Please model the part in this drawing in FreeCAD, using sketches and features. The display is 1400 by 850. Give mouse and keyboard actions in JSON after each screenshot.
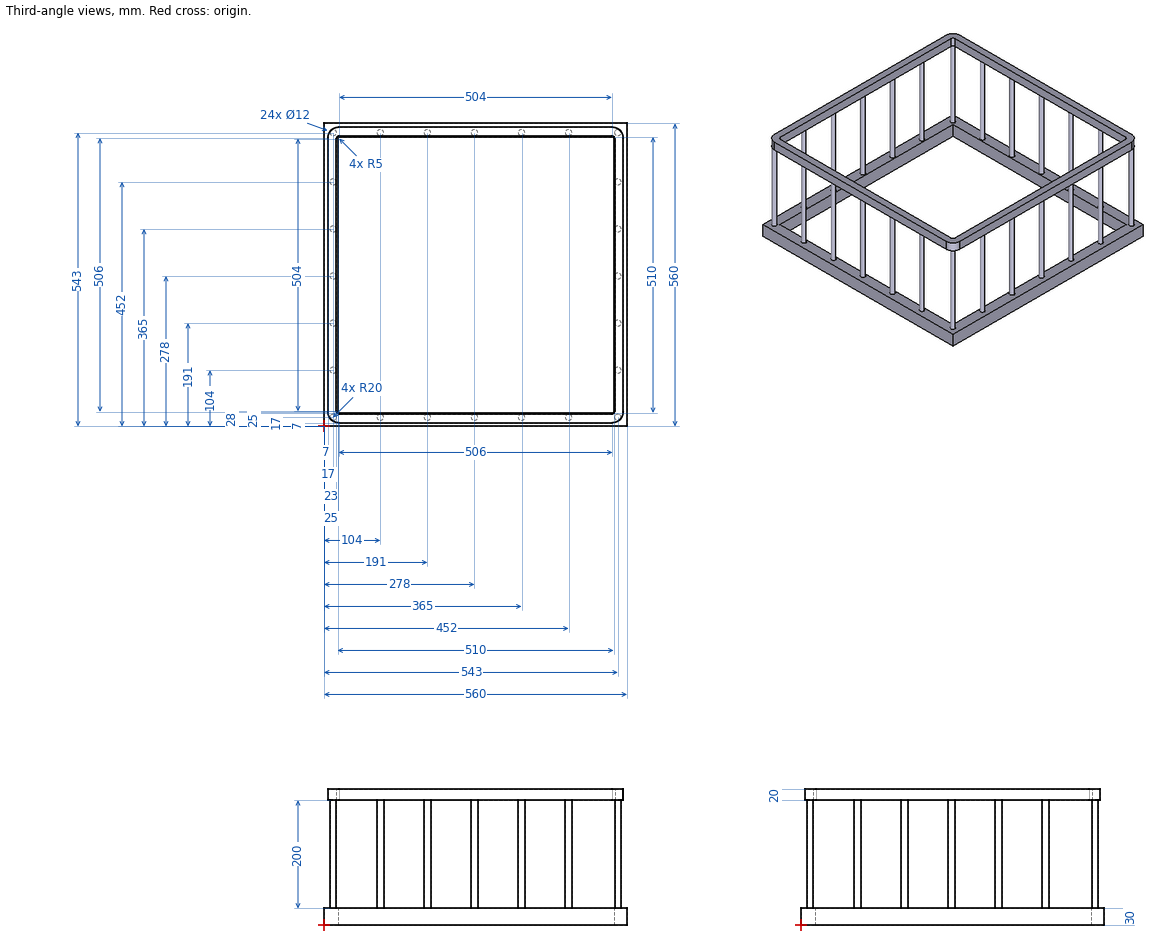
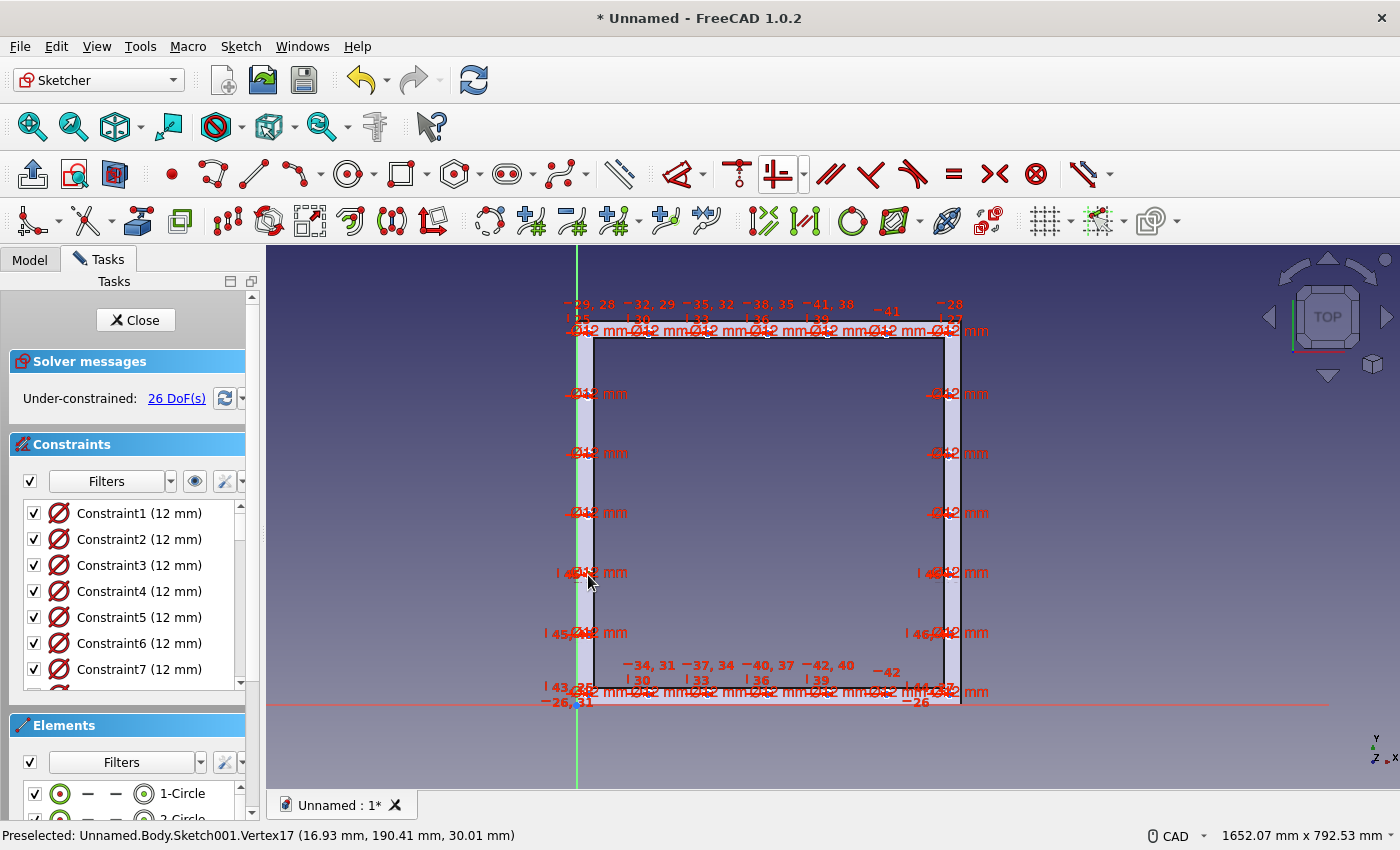
{"action": "left_click", "coordinate": [588, 515]}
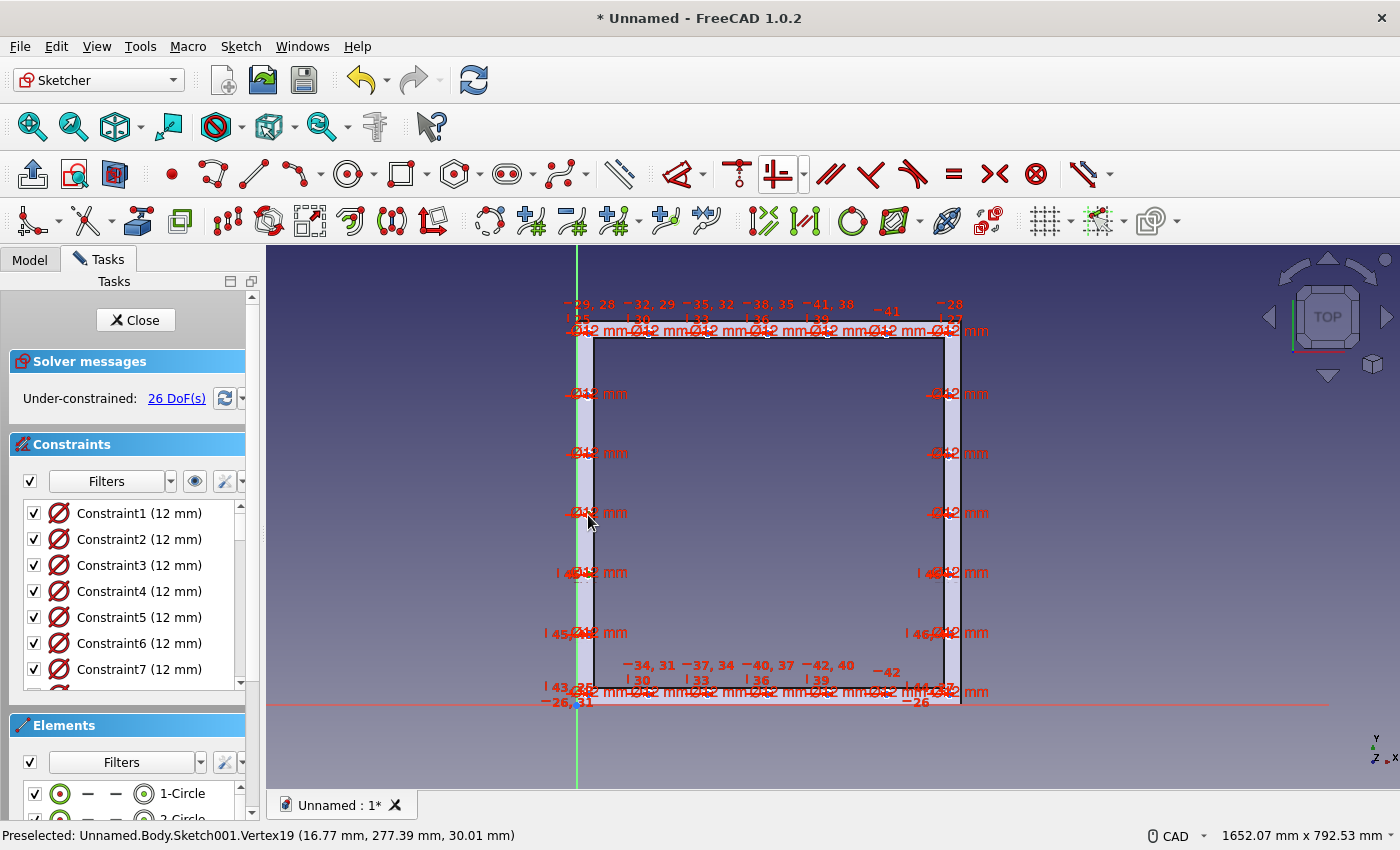
{"action": "key", "text": "v"}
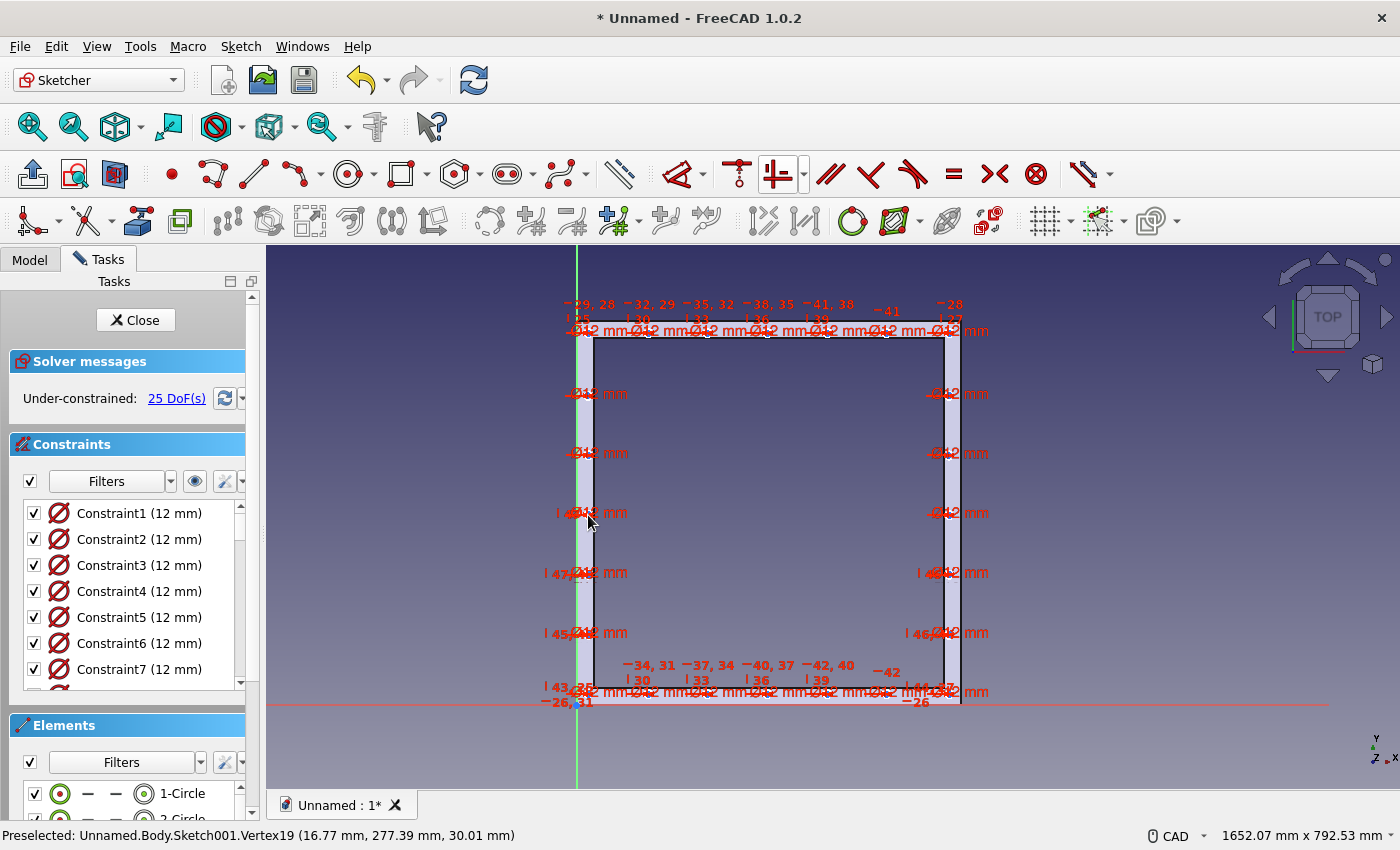
{"action": "left_click", "coordinate": [949, 575]}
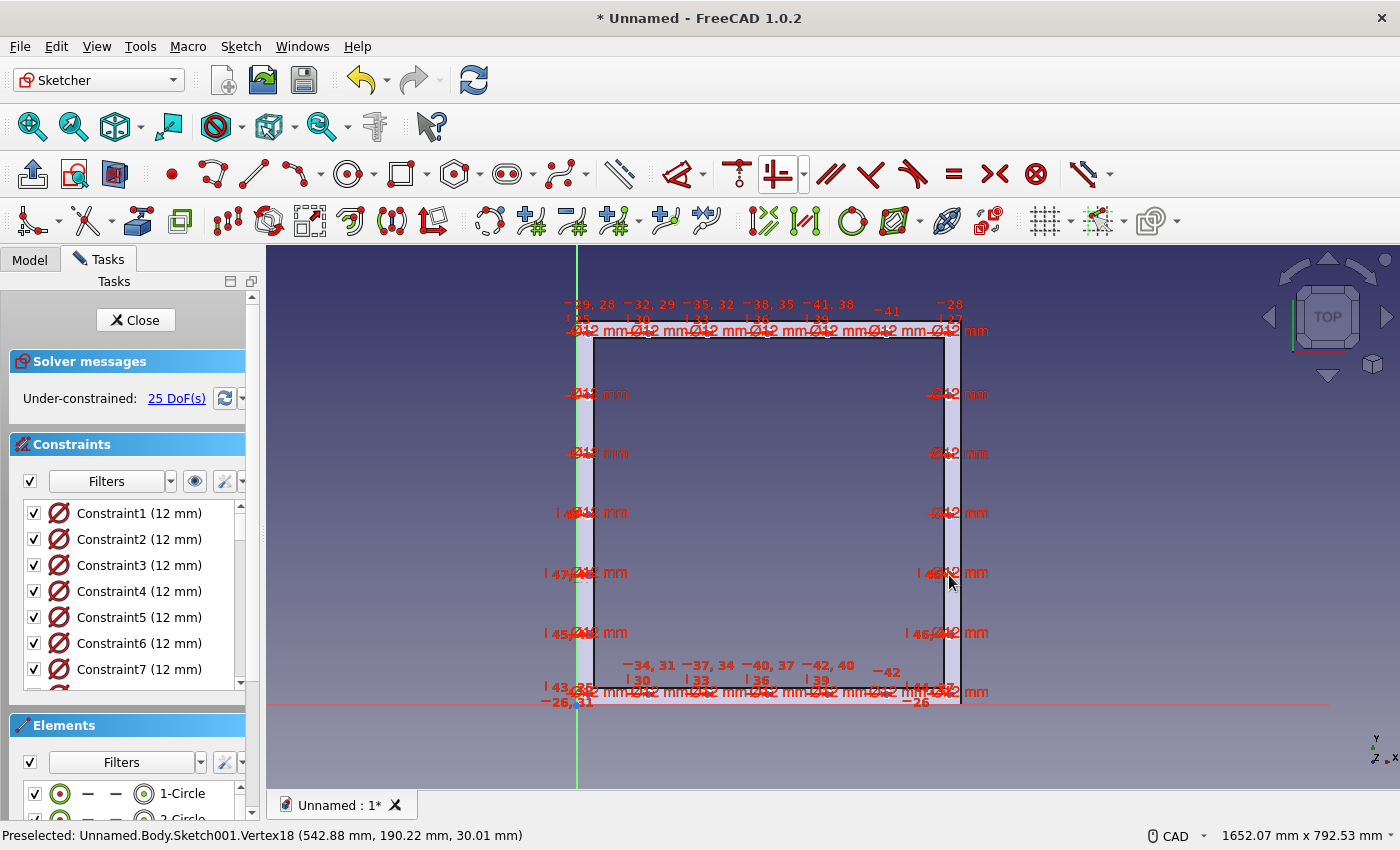
{"action": "left_click", "coordinate": [949, 515]}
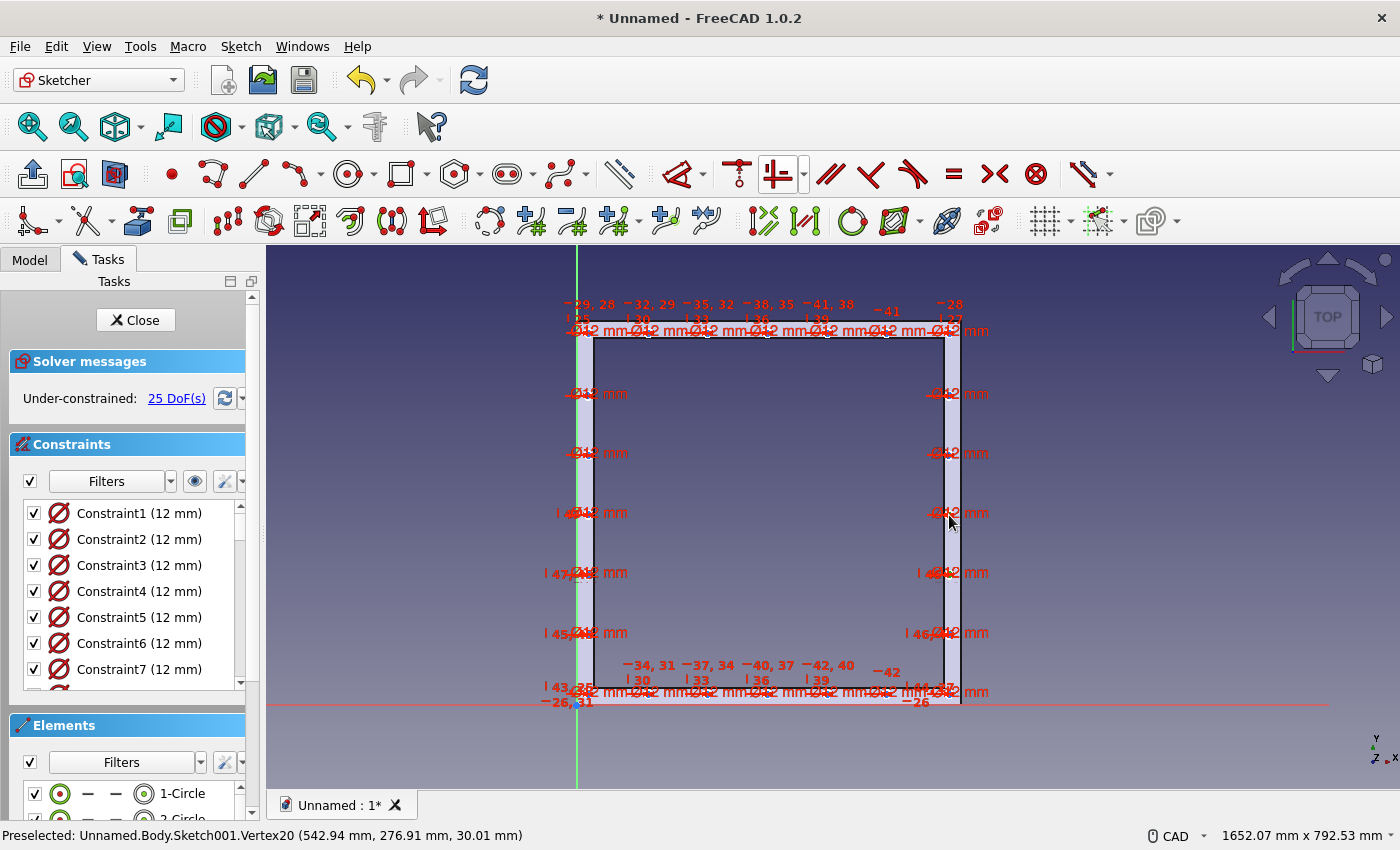
{"action": "key", "text": "v"}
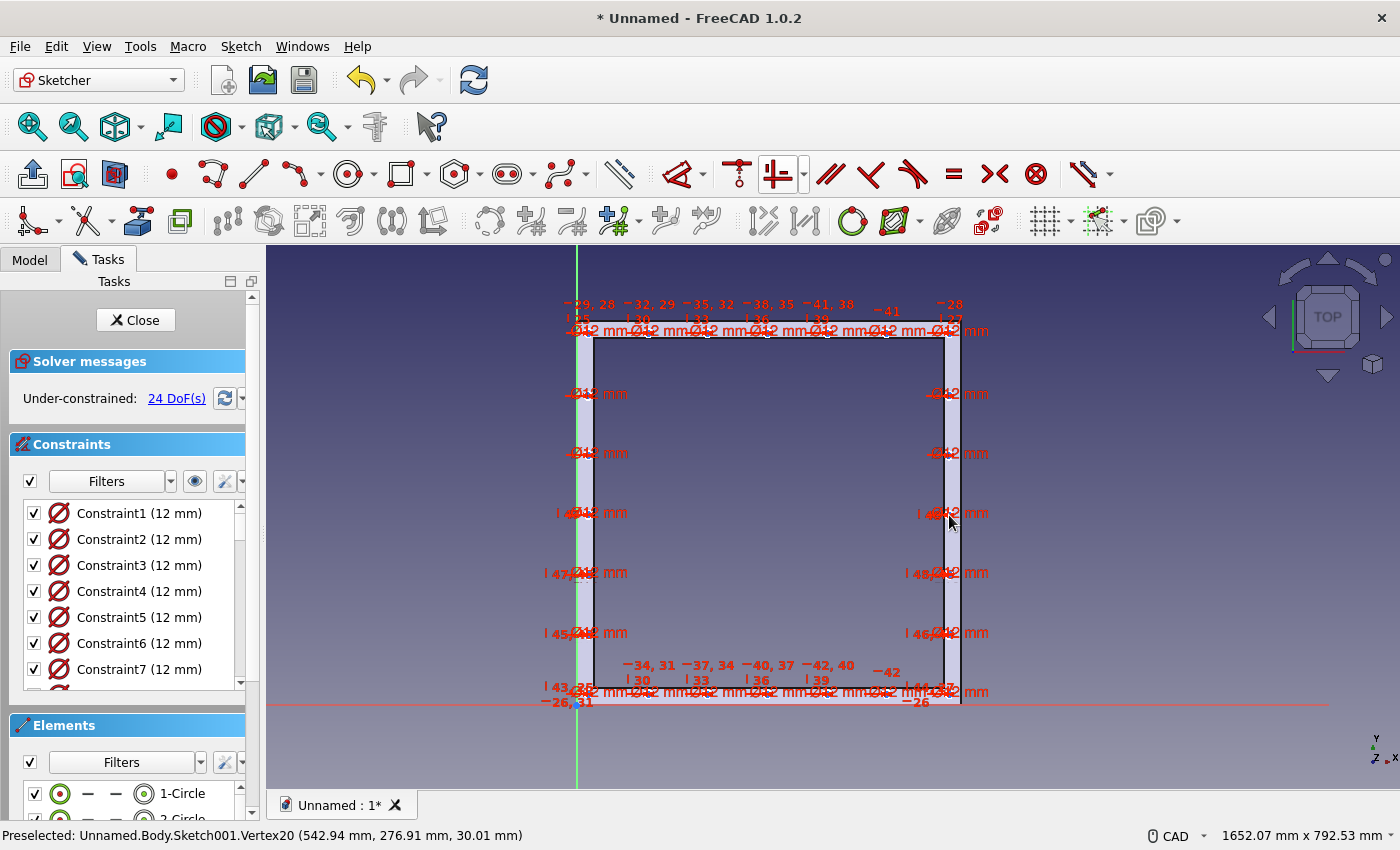
{"action": "left_click", "coordinate": [588, 515]}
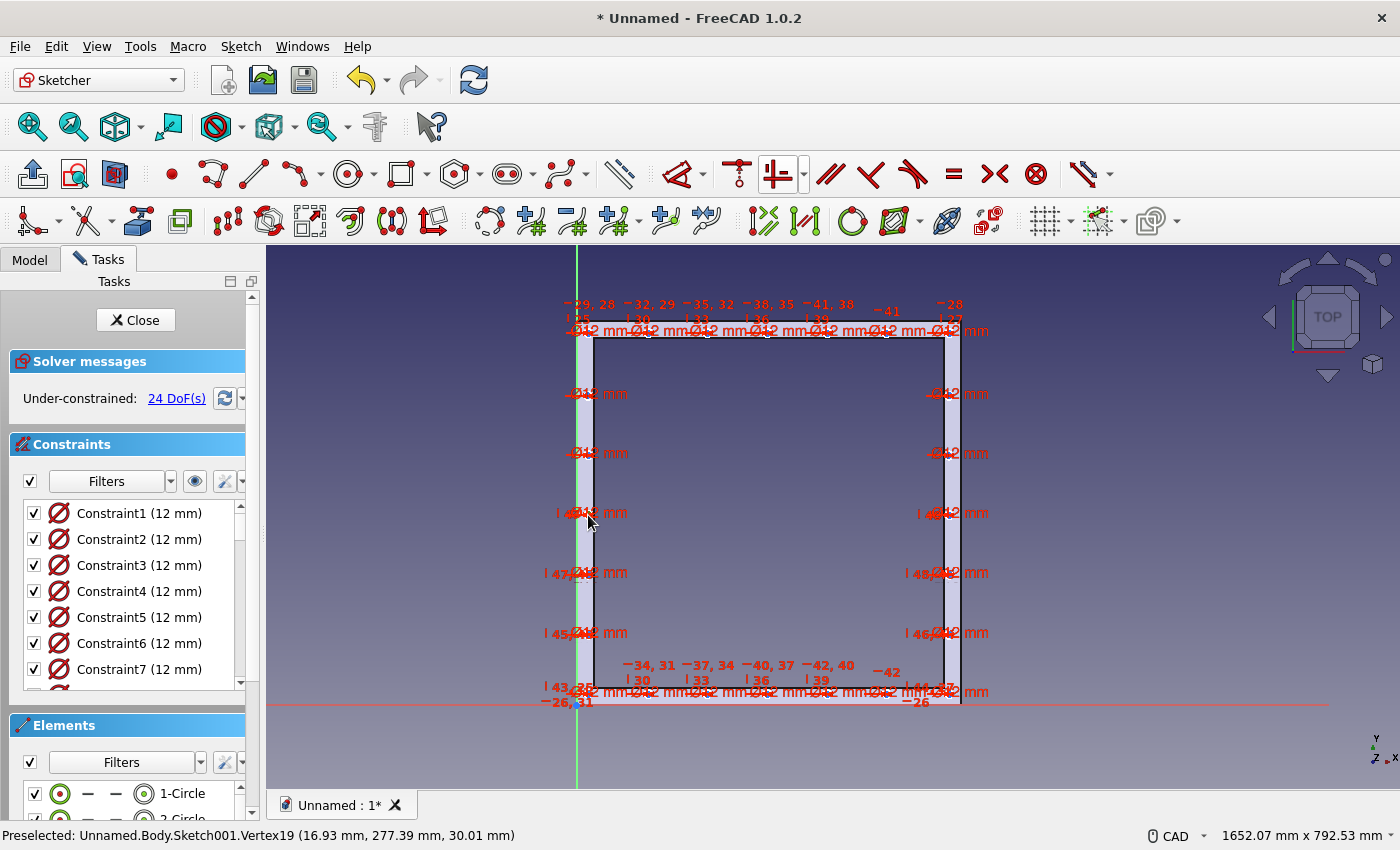
{"action": "left_click", "coordinate": [588, 455]}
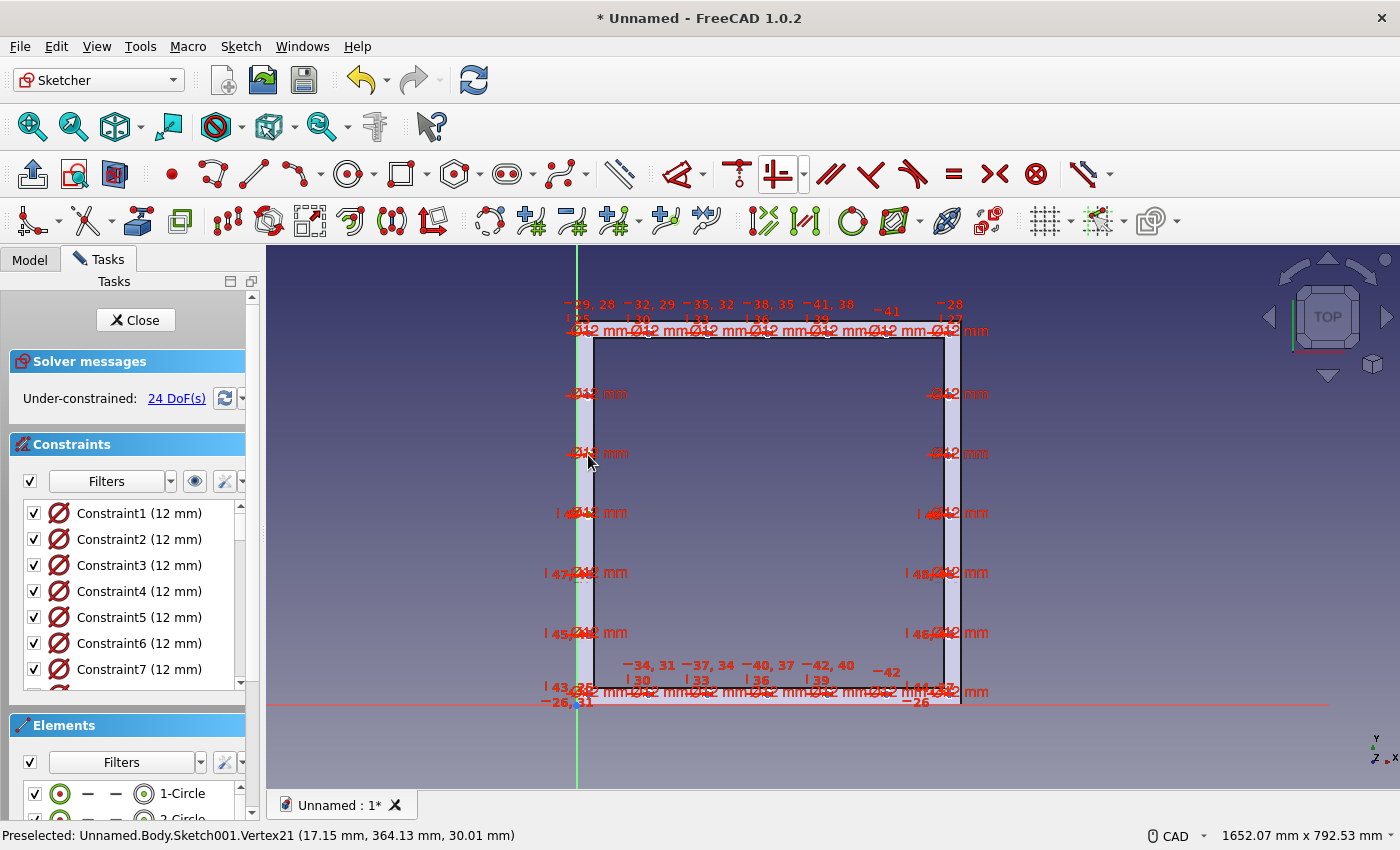
{"action": "key", "text": "v"}